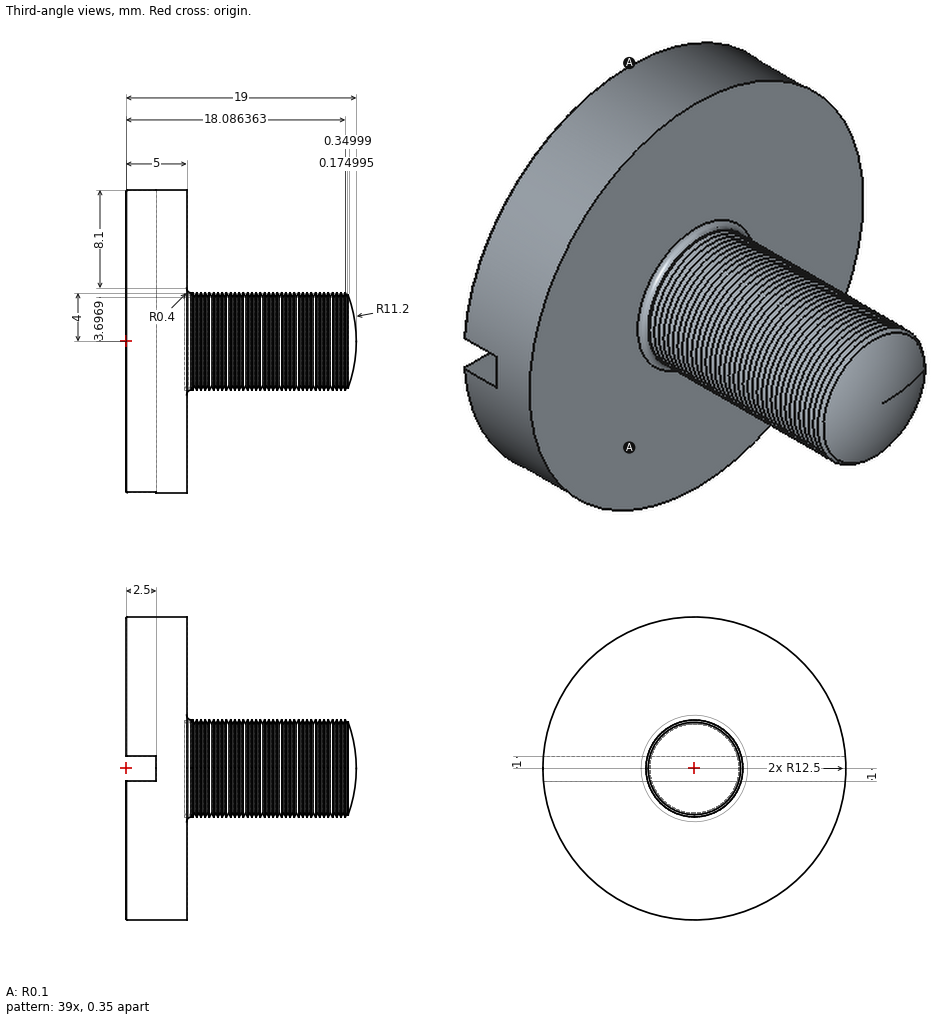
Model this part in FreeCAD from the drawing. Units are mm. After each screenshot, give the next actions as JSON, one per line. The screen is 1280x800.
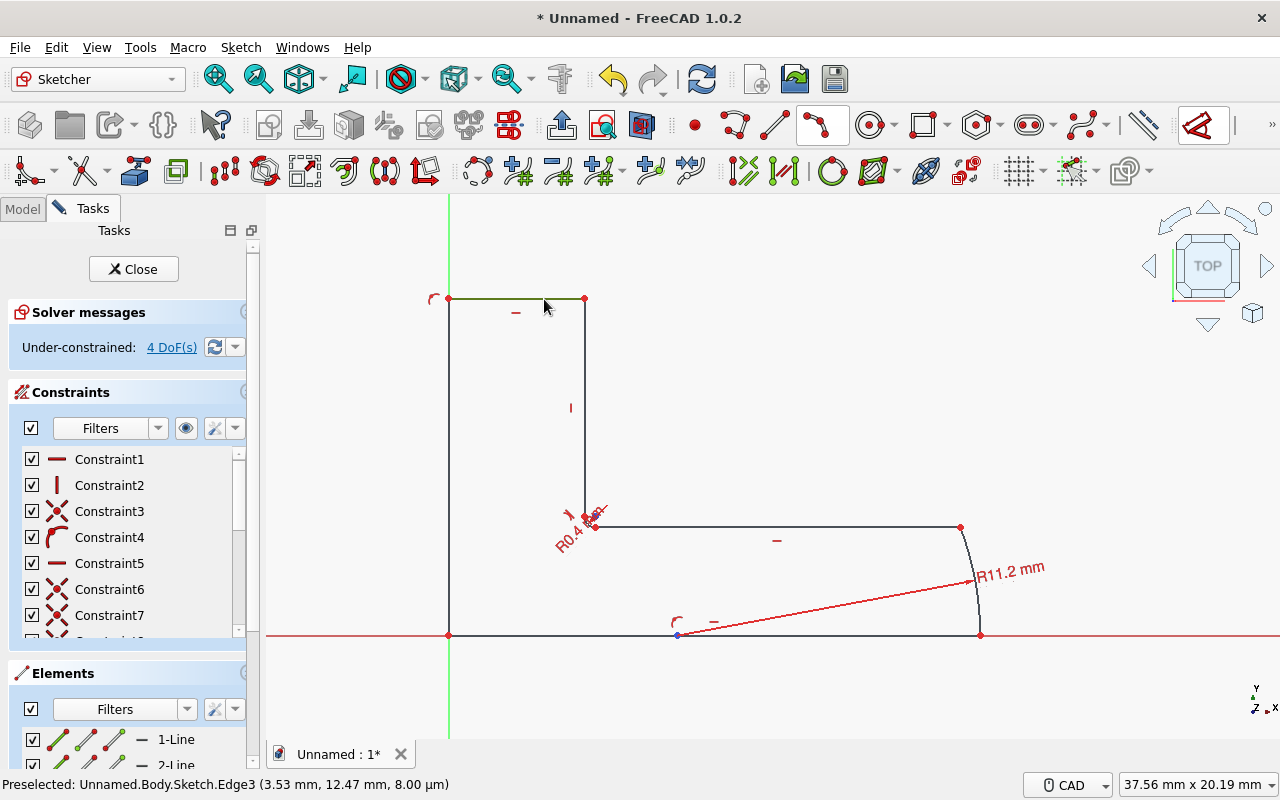
{"action": "key", "text": "l"}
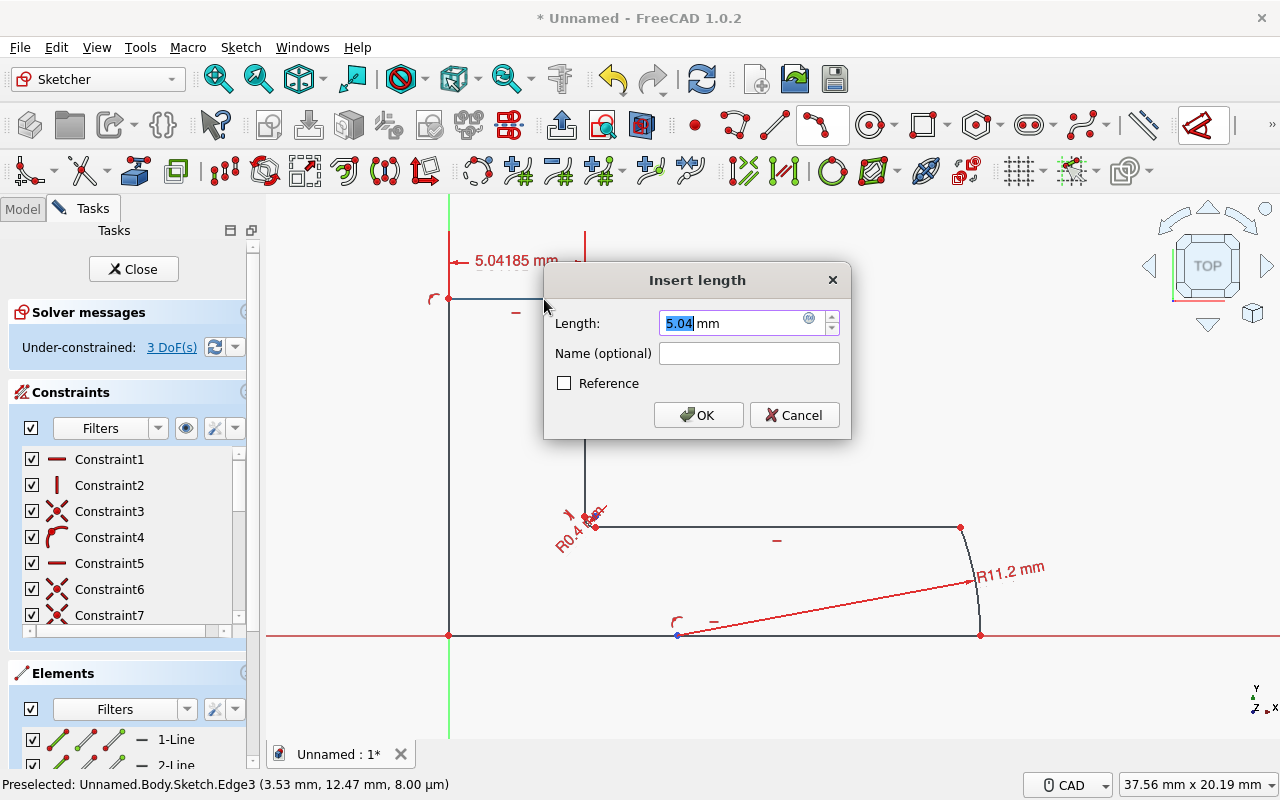
{"action": "type", "text": "5"}
{"action": "key", "text": "Return"}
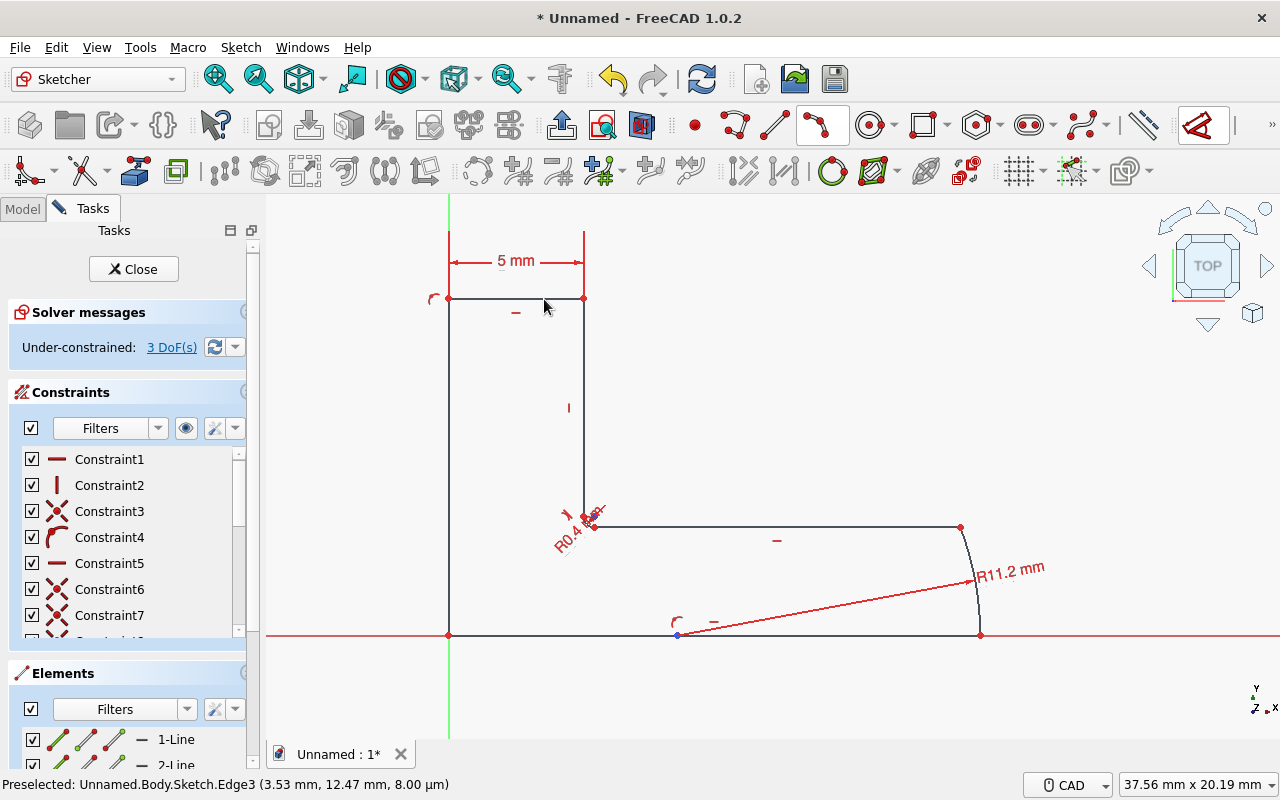
{"action": "left_click", "coordinate": [608, 636]}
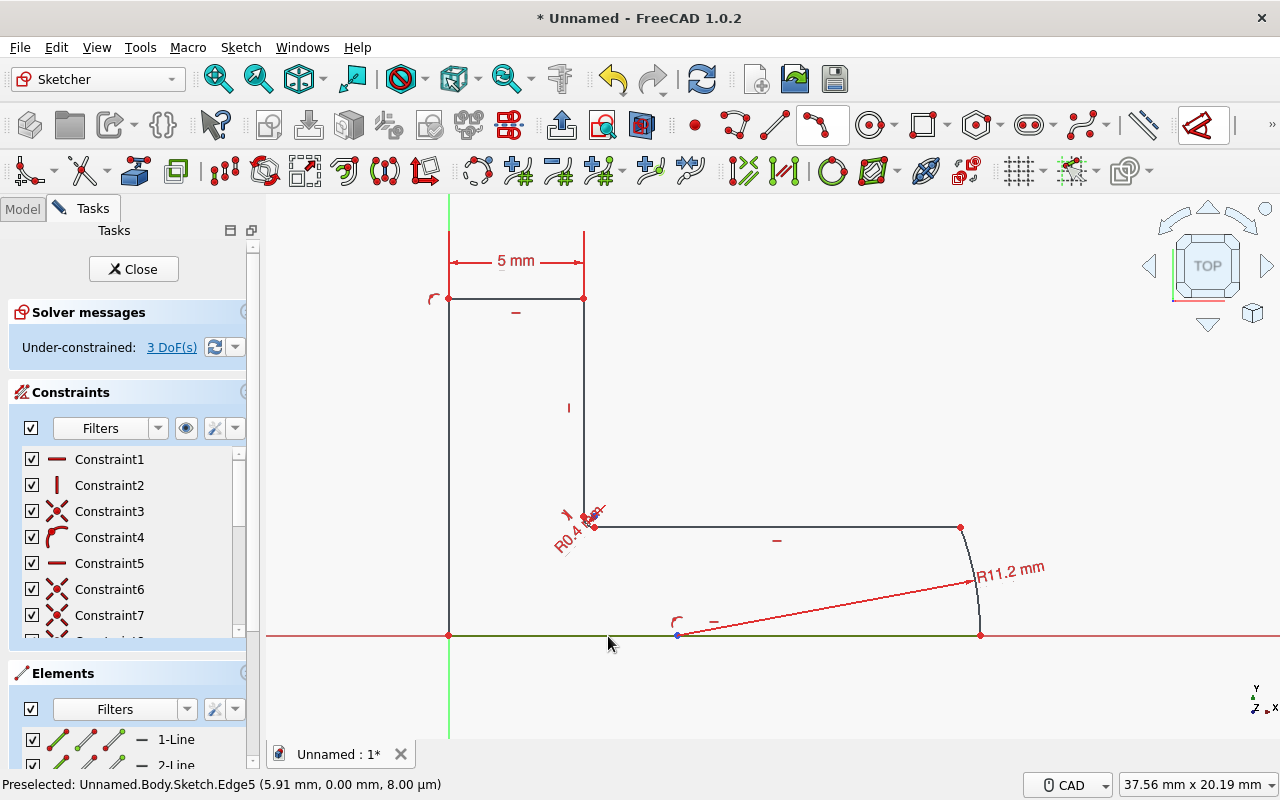
{"action": "left_click", "coordinate": [1224, 126]}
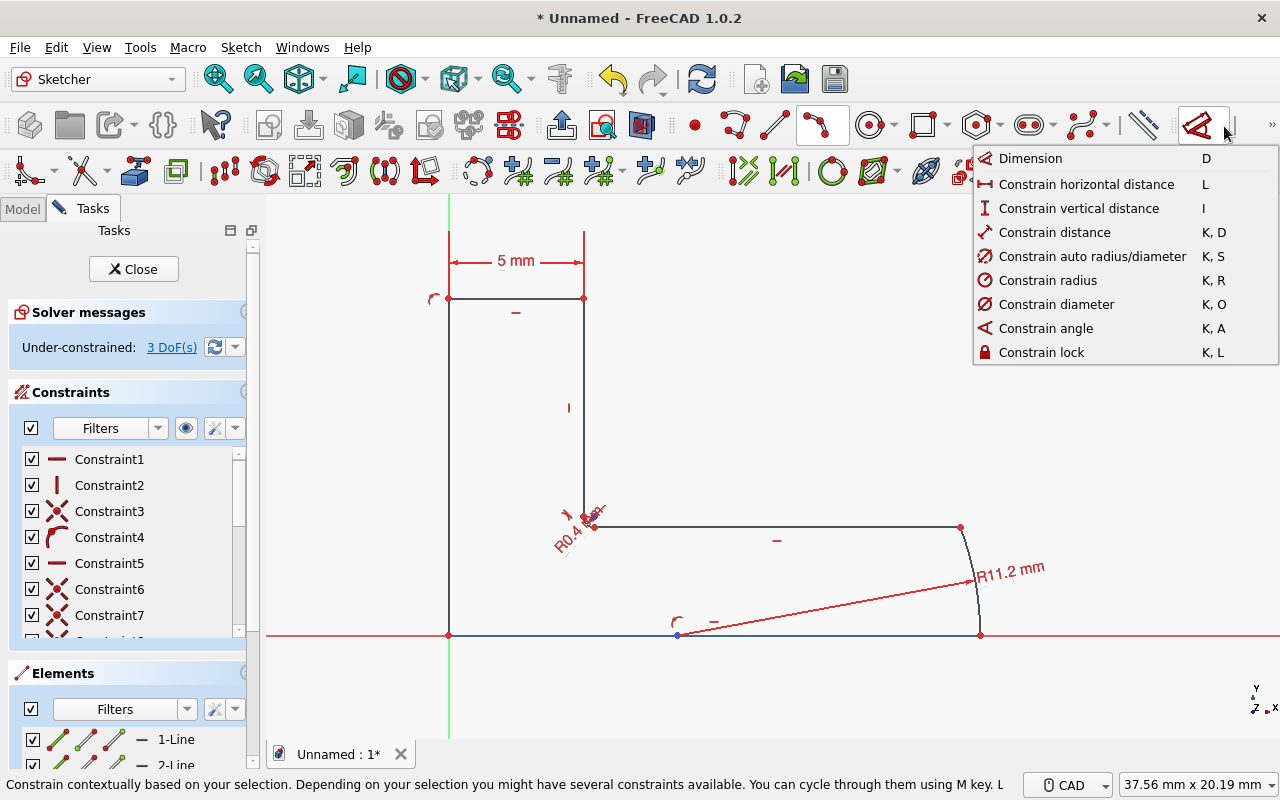
{"action": "left_click", "coordinate": [1126, 184]}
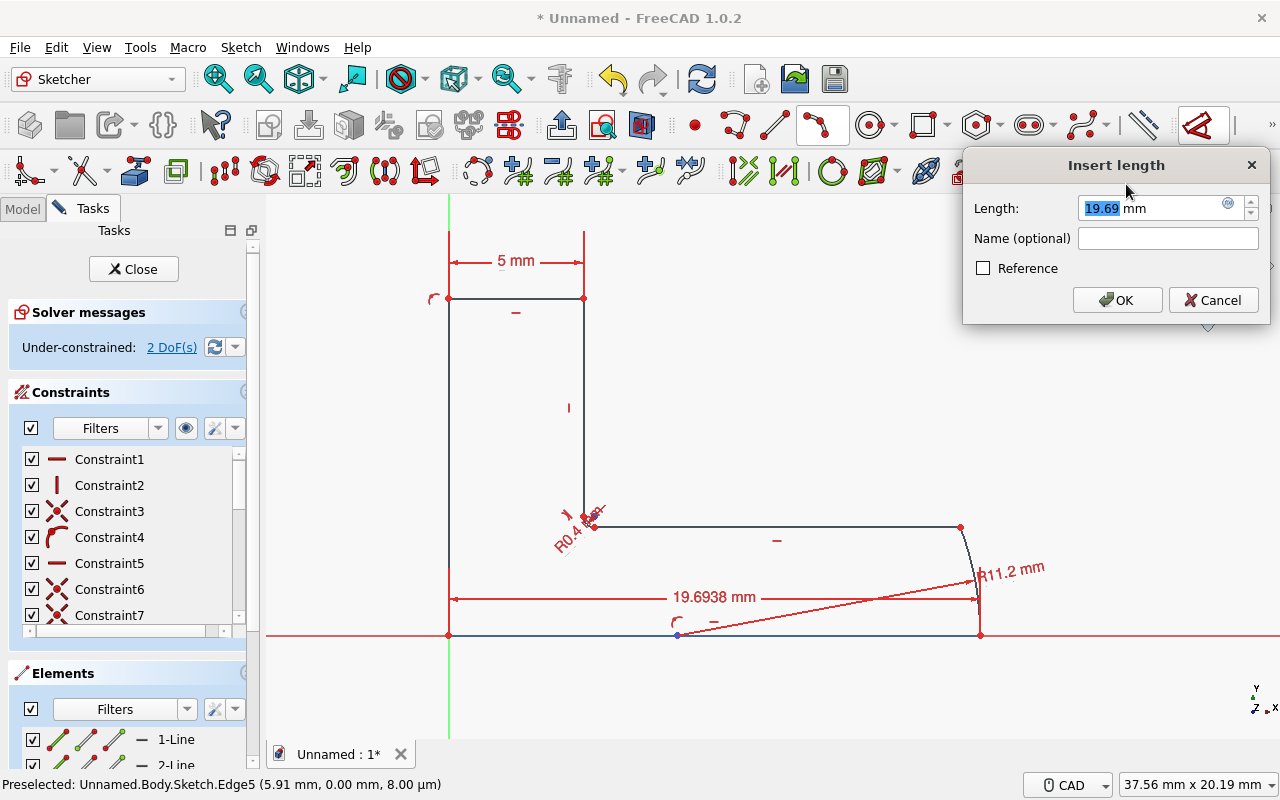
{"action": "type", "text": "19"}
{"action": "key", "text": "Return"}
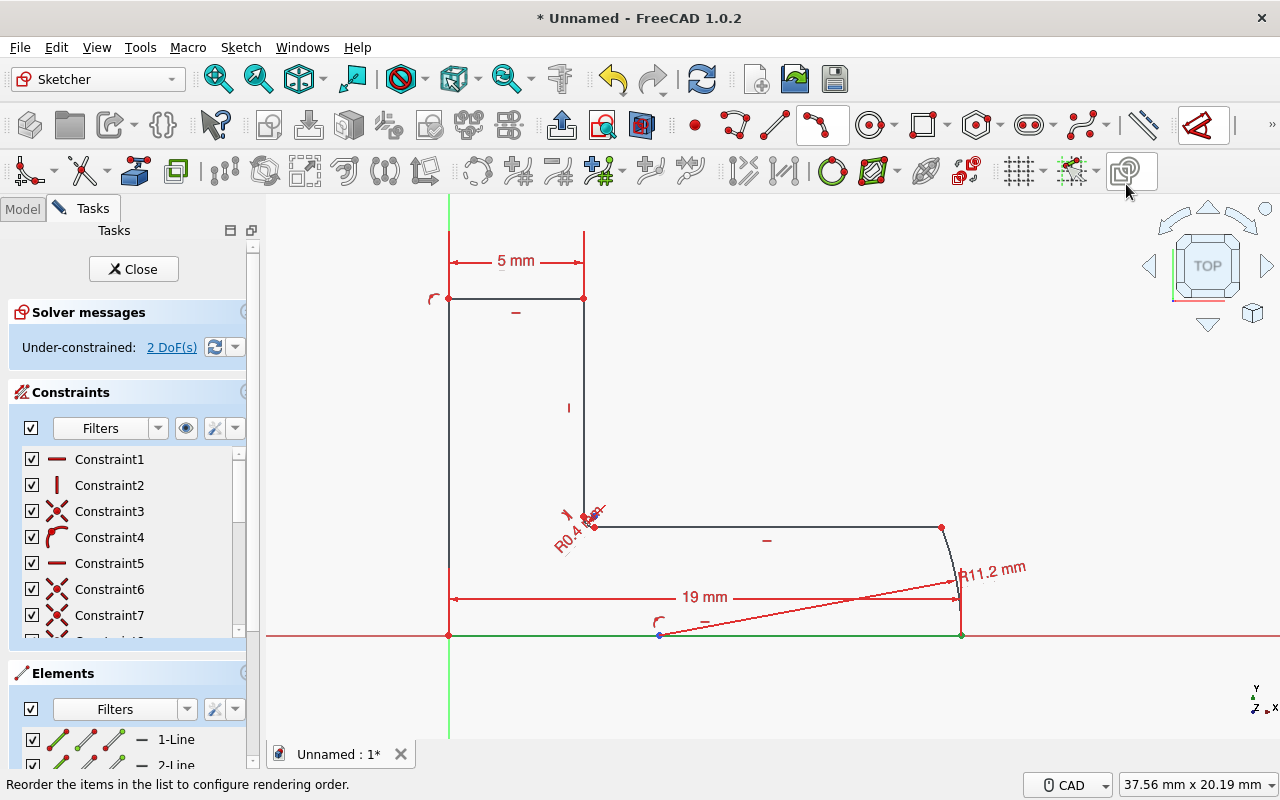
{"action": "left_click", "coordinate": [941, 527]}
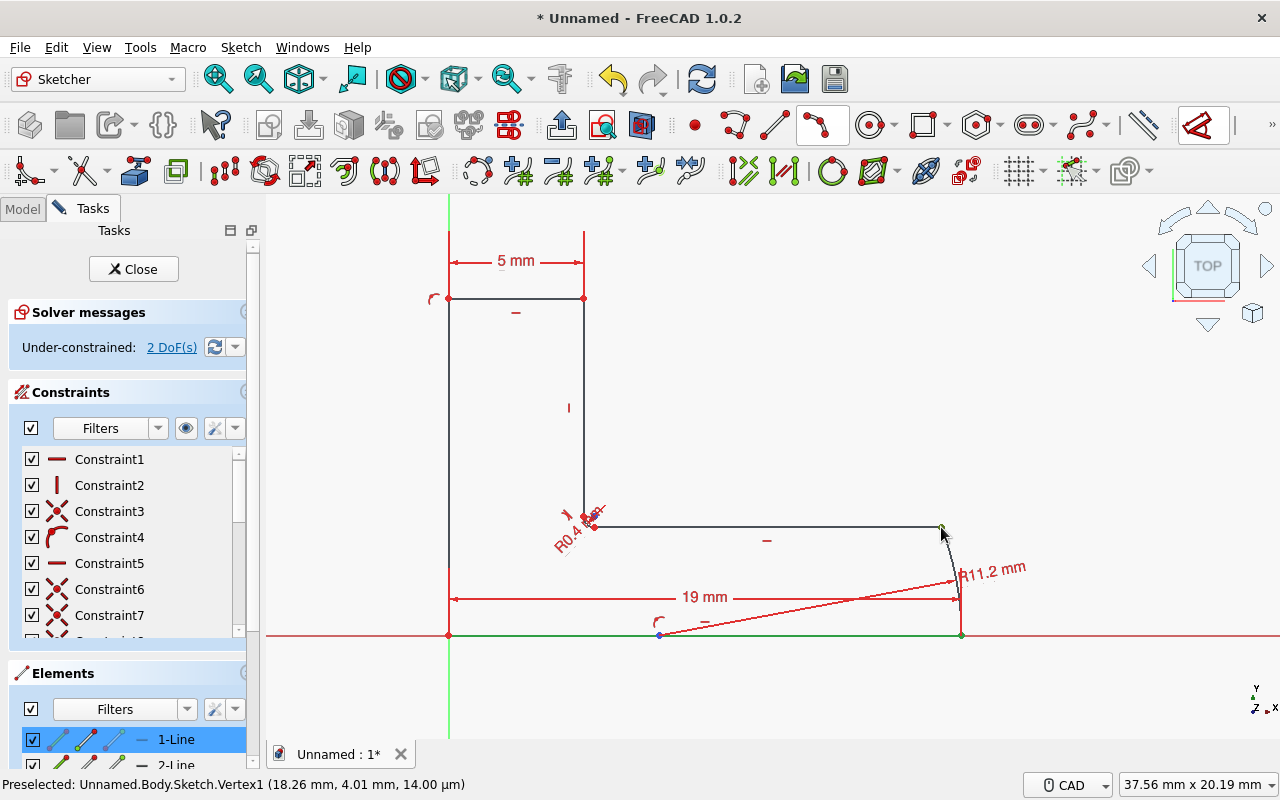
{"action": "key", "text": "i"}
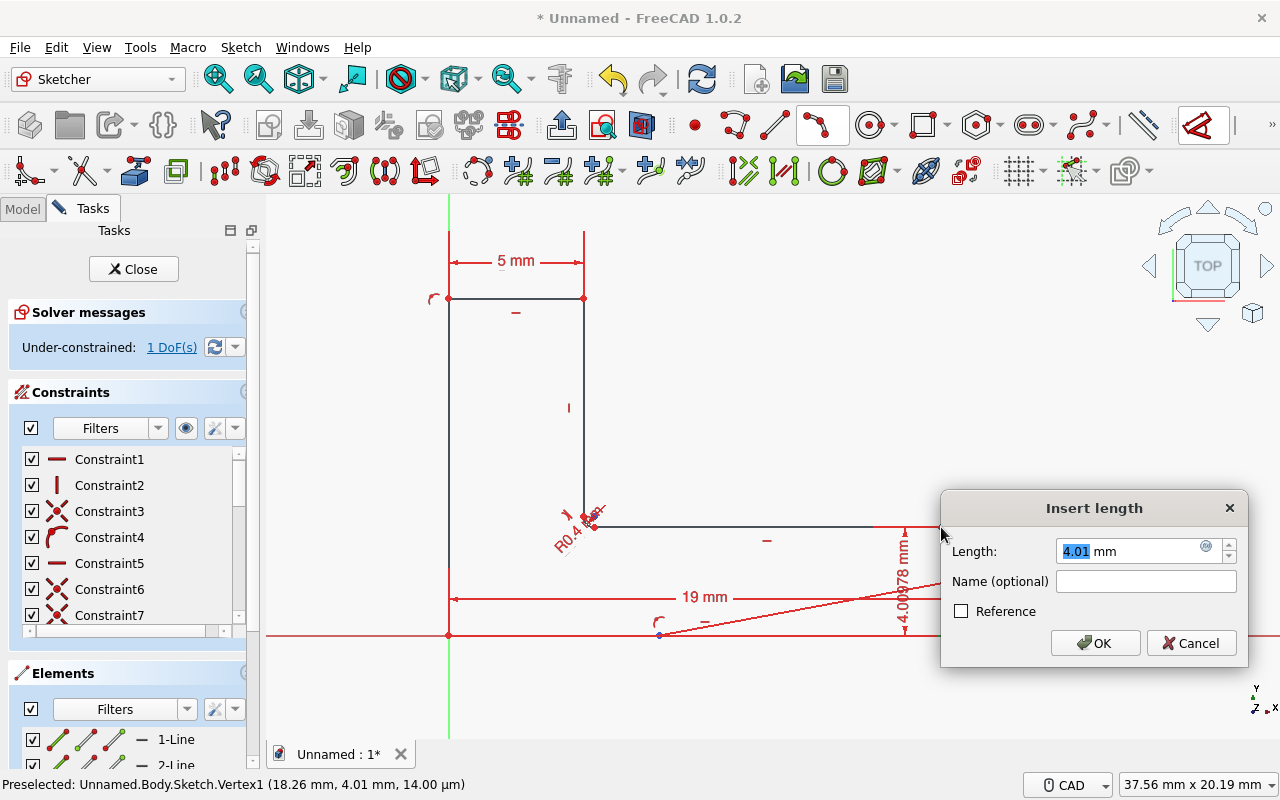
{"action": "type", "text": "4"}
{"action": "key", "text": "Return"}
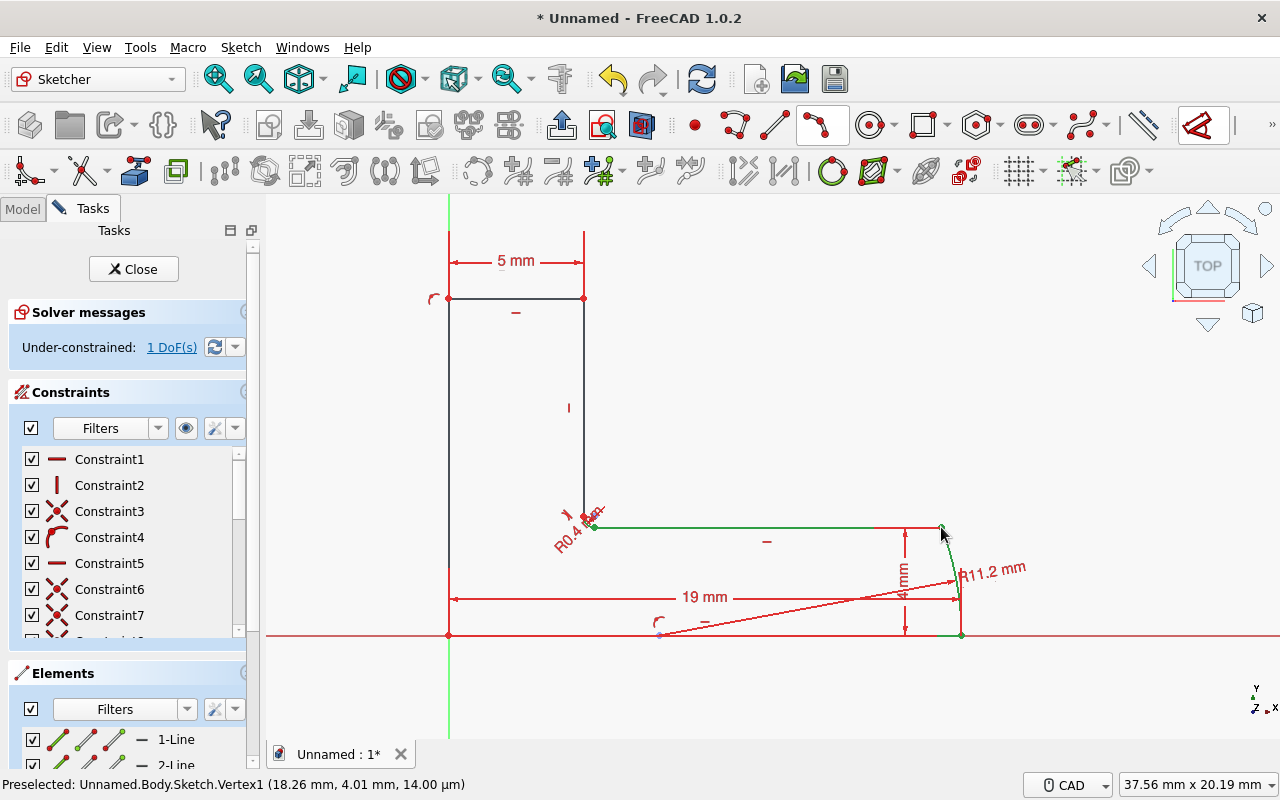
{"action": "left_click", "coordinate": [584, 451]}